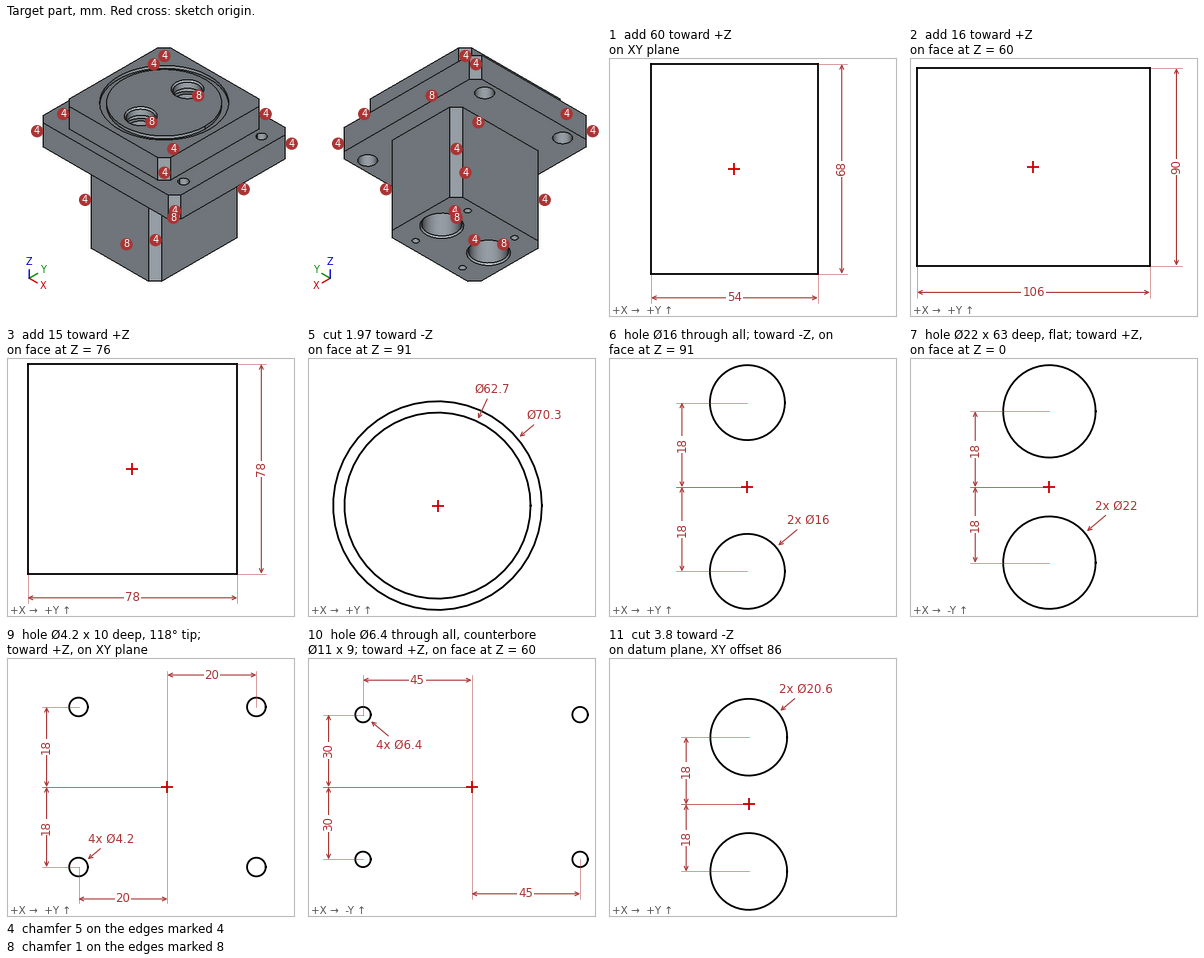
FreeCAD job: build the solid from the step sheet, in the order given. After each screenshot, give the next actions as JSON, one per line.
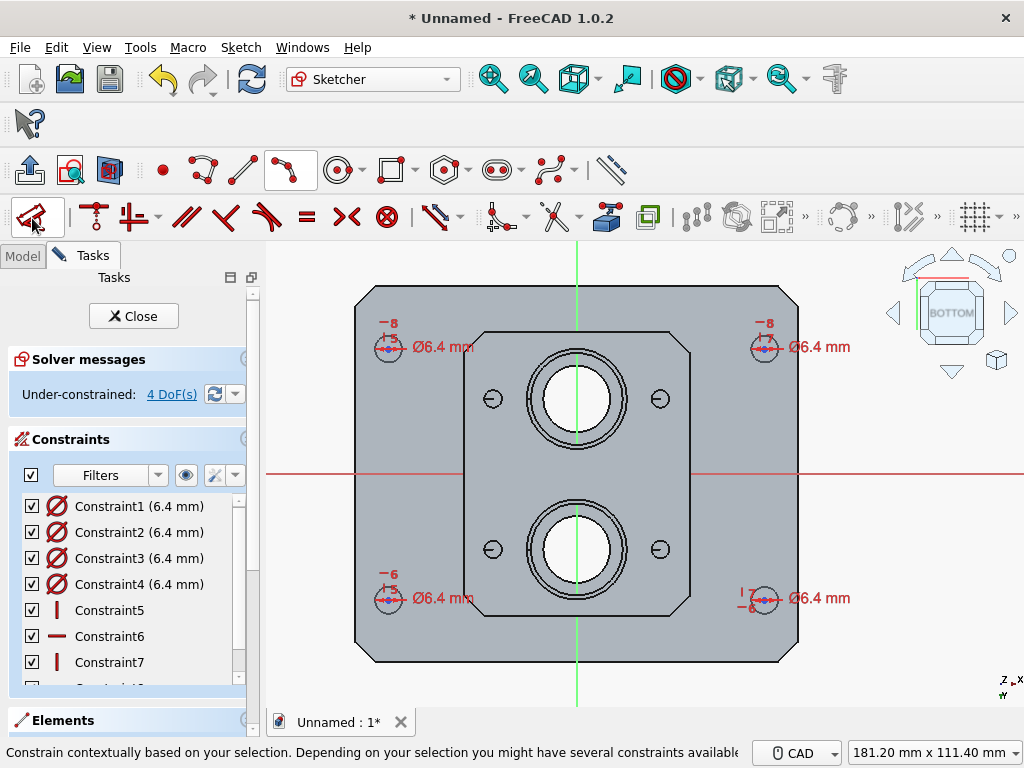
{"action": "left_click", "coordinate": [389, 349]}
{"action": "left_click", "coordinate": [483, 315]}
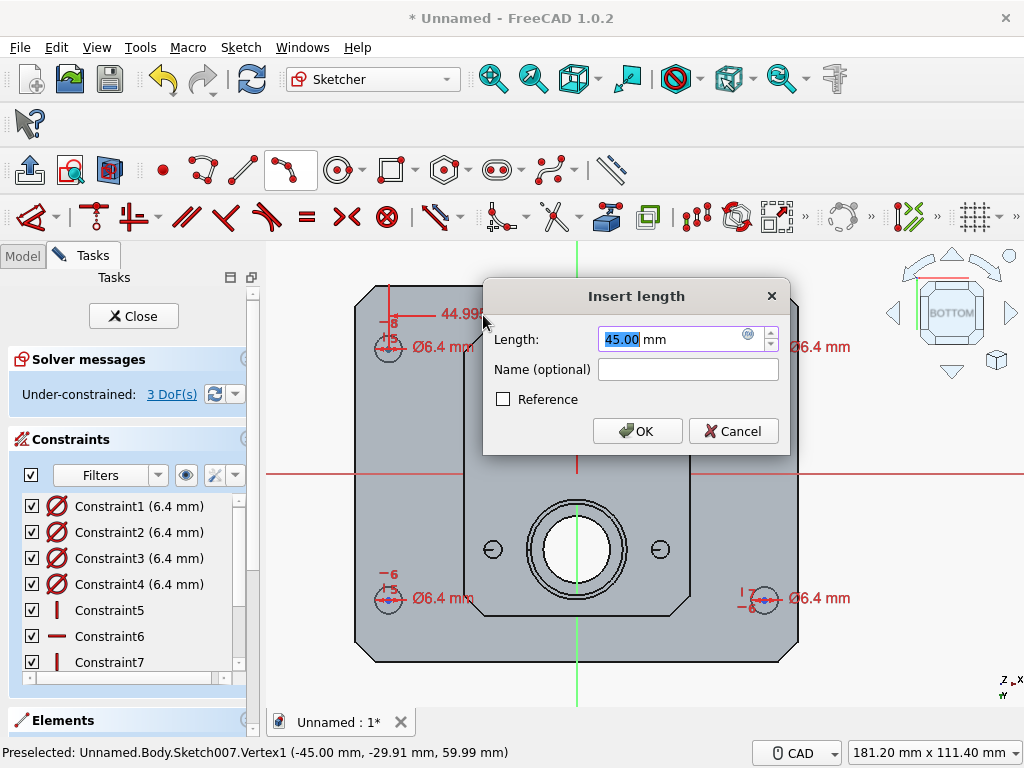
{"action": "type", "text": "45"}
{"action": "key", "text": "Return"}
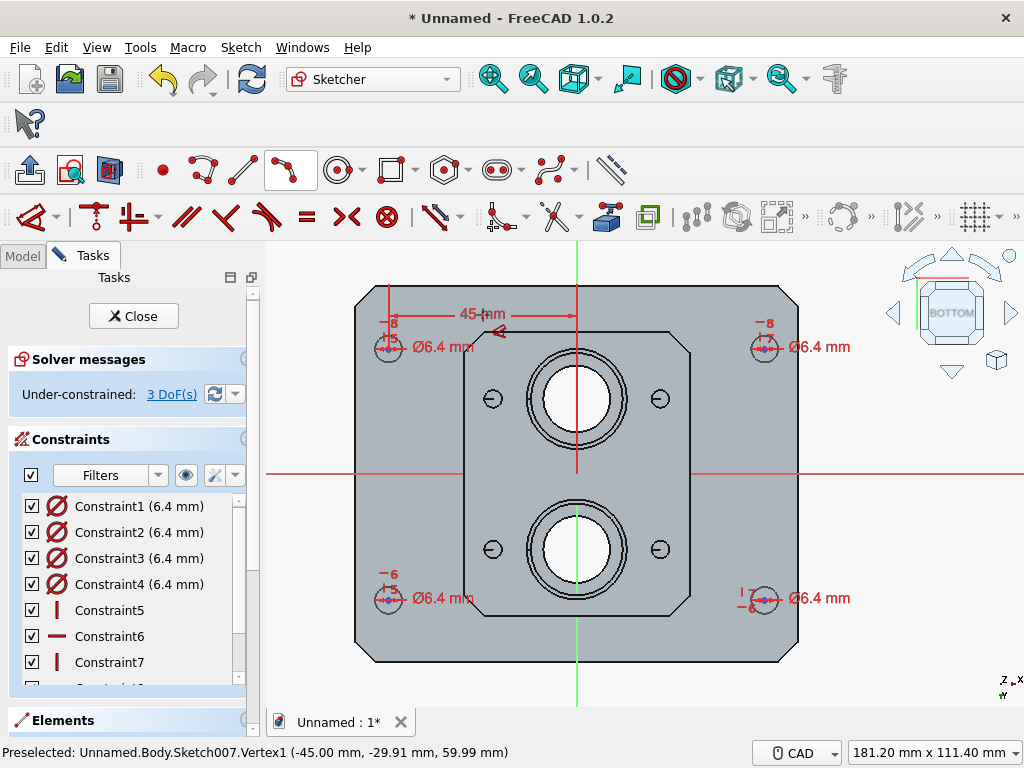
{"action": "left_click", "coordinate": [389, 349]}
{"action": "left_click", "coordinate": [355, 412]}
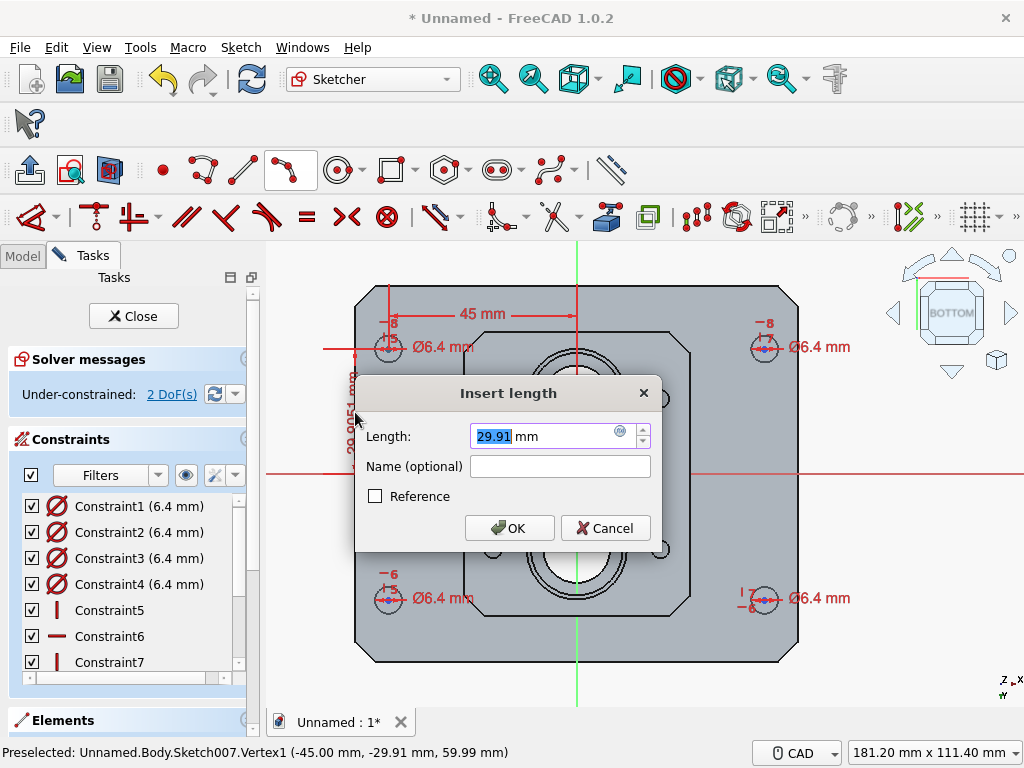
{"action": "type", "text": "30"}
{"action": "key", "text": "Return"}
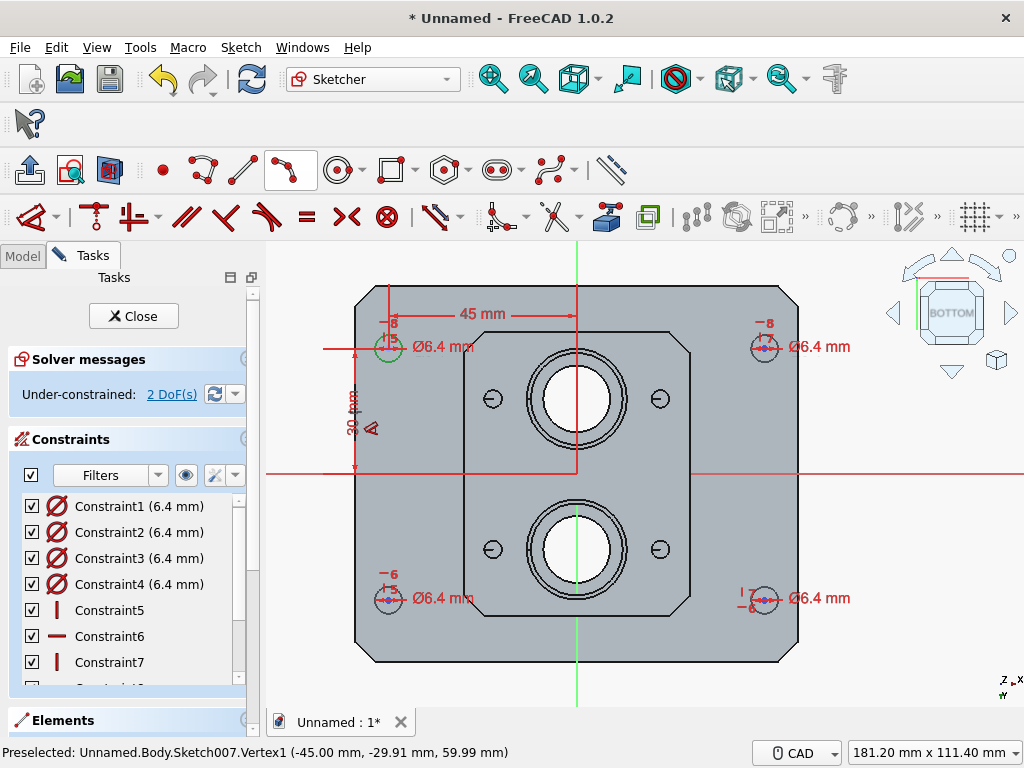
{"action": "left_click", "coordinate": [389, 600]}
{"action": "left_click", "coordinate": [355, 537]}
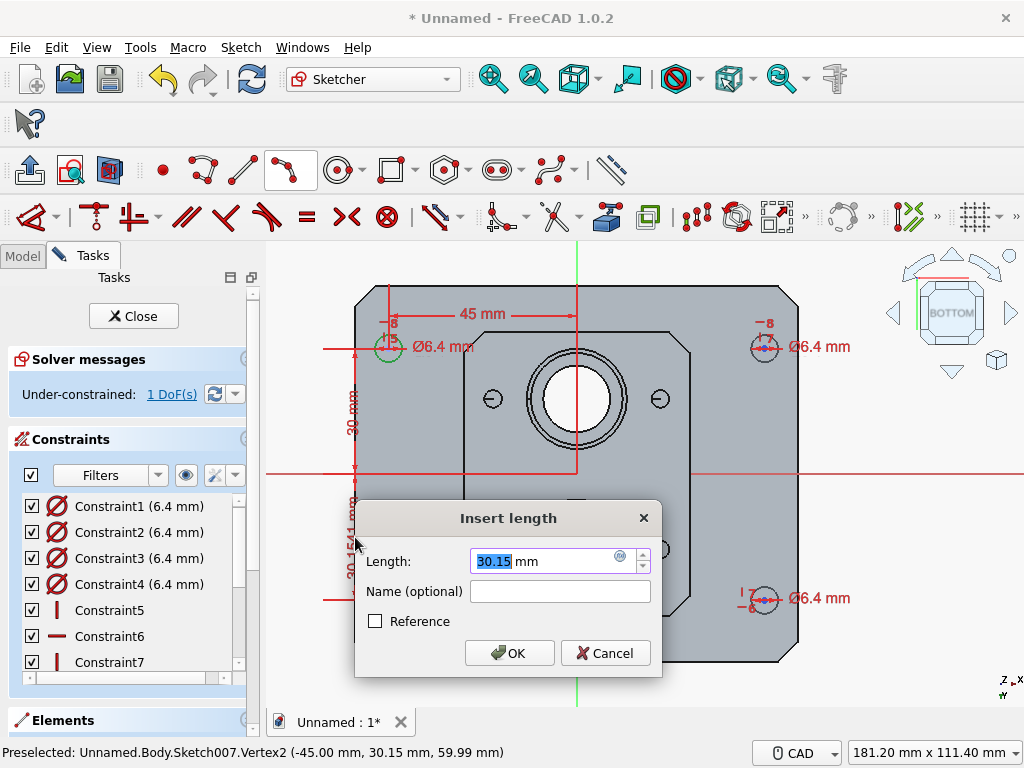
{"action": "type", "text": "30"}
{"action": "key", "text": "Return"}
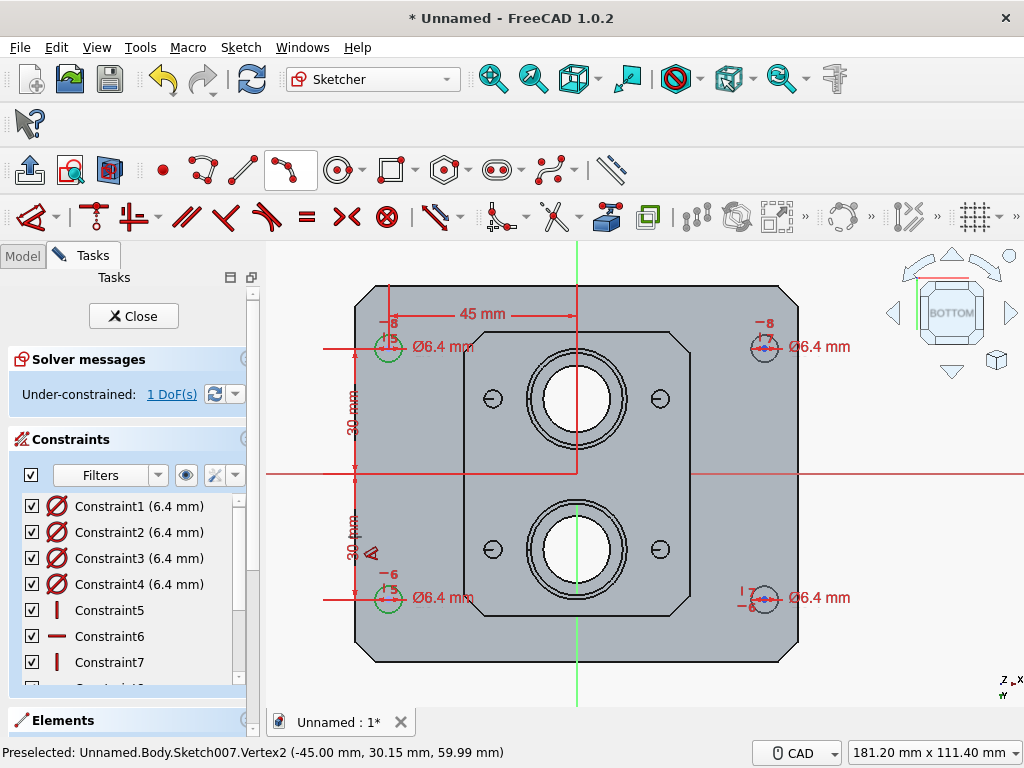
{"action": "left_click", "coordinate": [765, 600]}
{"action": "left_click", "coordinate": [671, 634]}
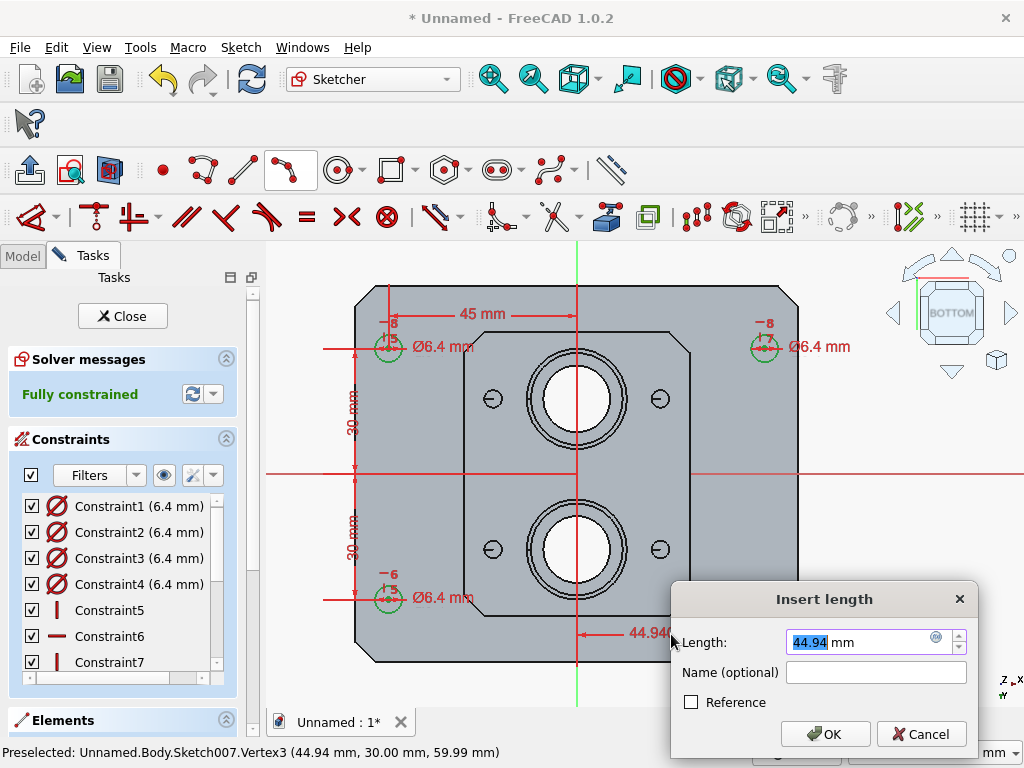
{"action": "type", "text": "45"}
{"action": "key", "text": "Return"}
{"action": "key", "text": "Escape"}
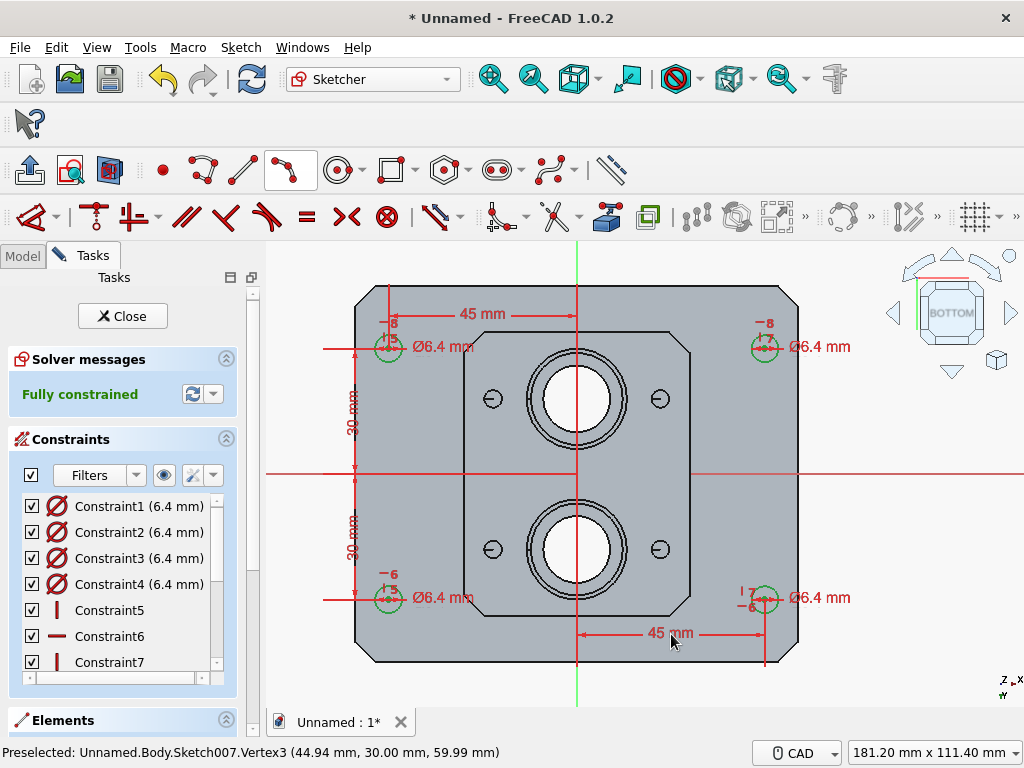
{"action": "left_click", "coordinate": [123, 316]}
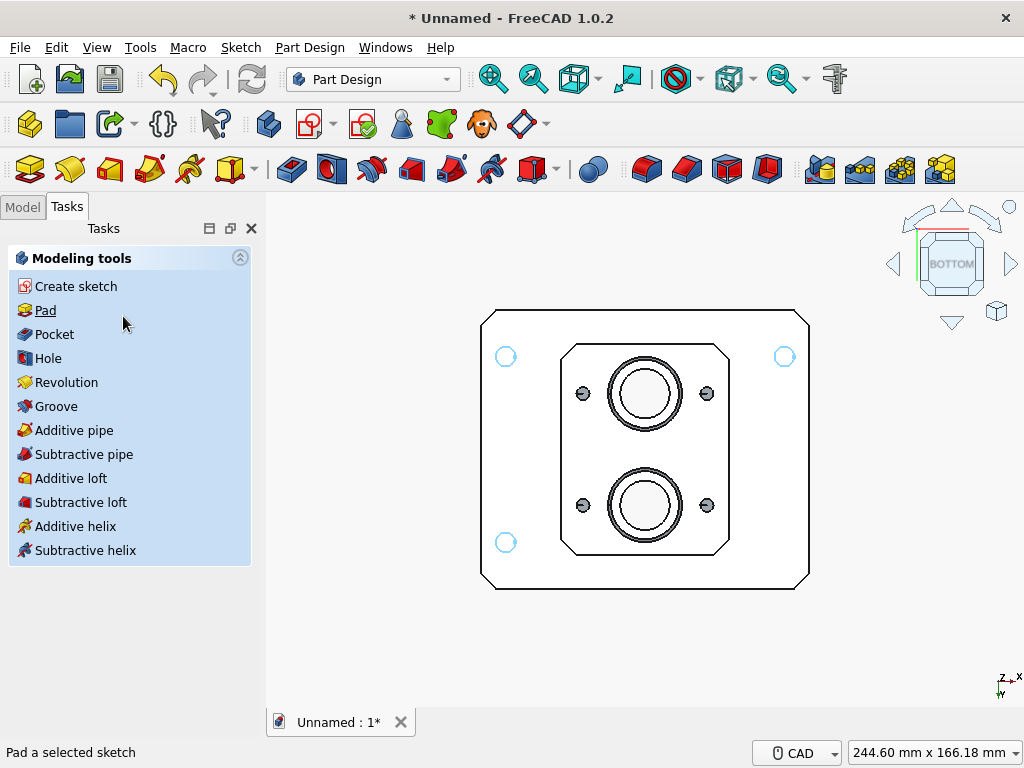
{"action": "left_click", "coordinate": [332, 170]}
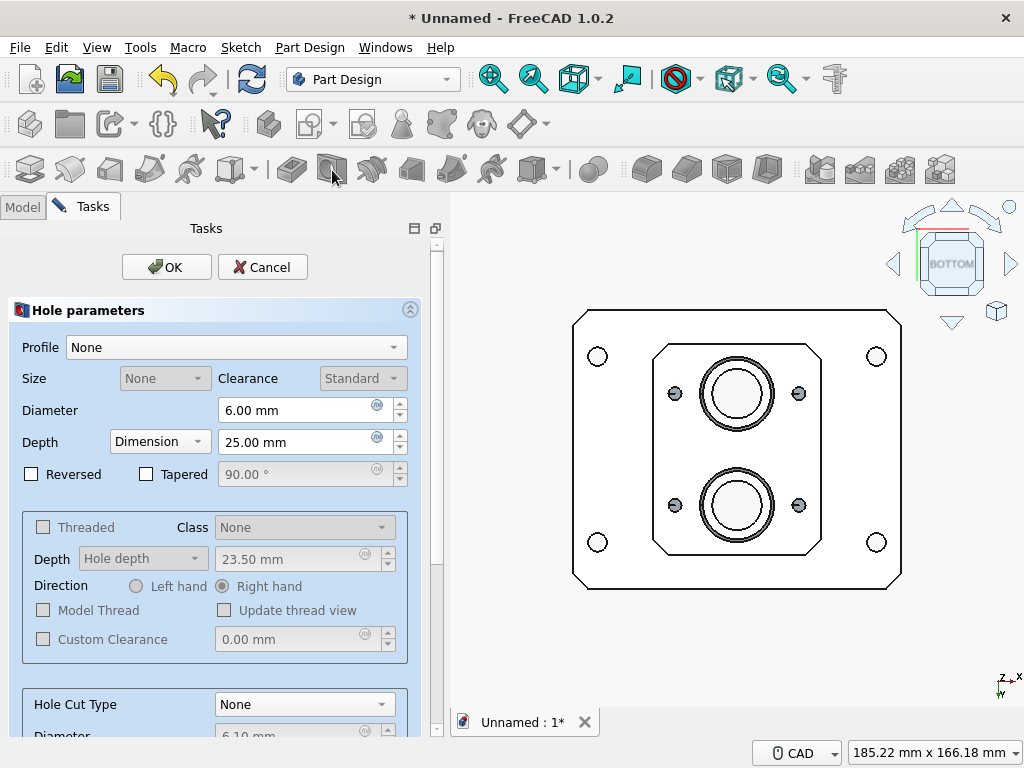
{"action": "triple_click", "coordinate": [305, 410]}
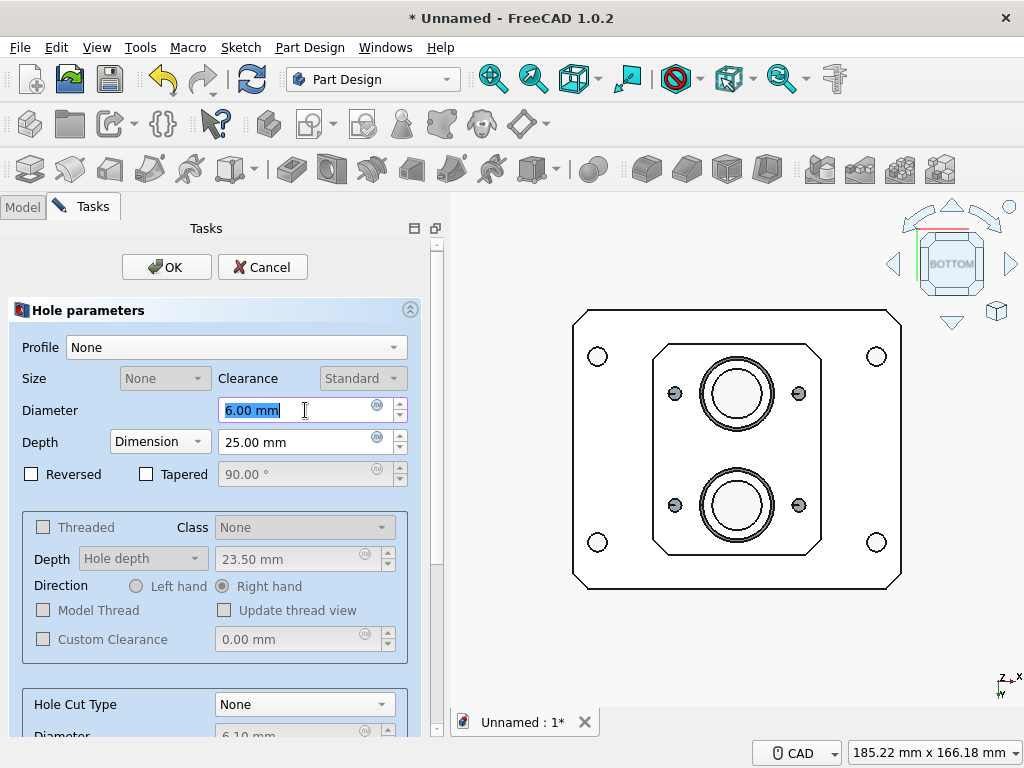
{"action": "type", "text": "6.4"}
{"action": "key", "text": "Tab"}